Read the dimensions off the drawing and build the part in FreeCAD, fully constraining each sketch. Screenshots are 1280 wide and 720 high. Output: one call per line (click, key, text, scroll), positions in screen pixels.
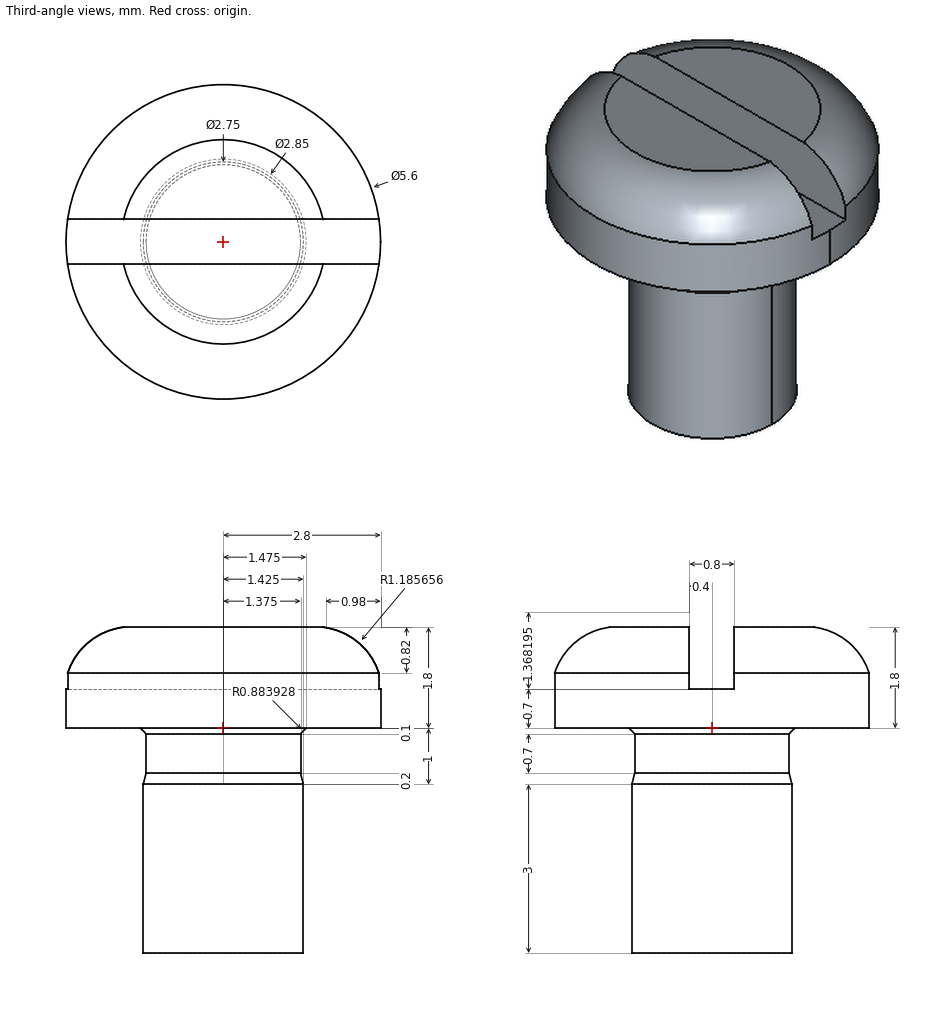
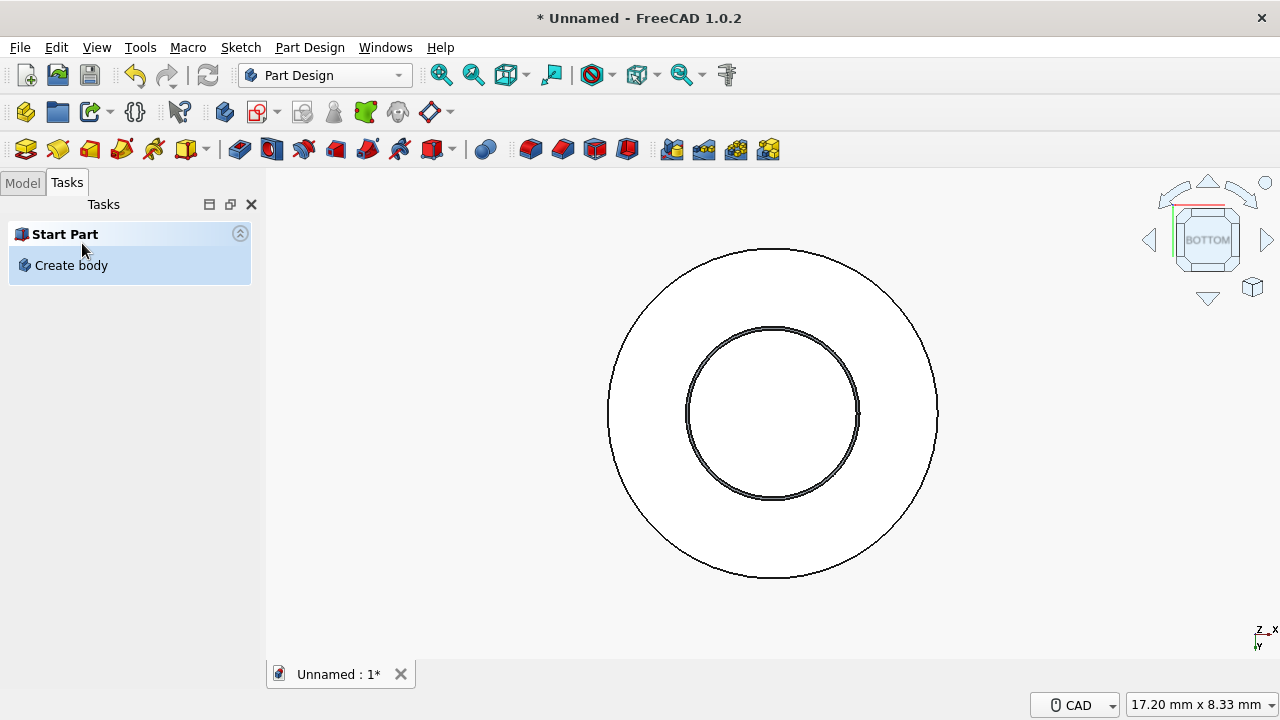
click(773, 412)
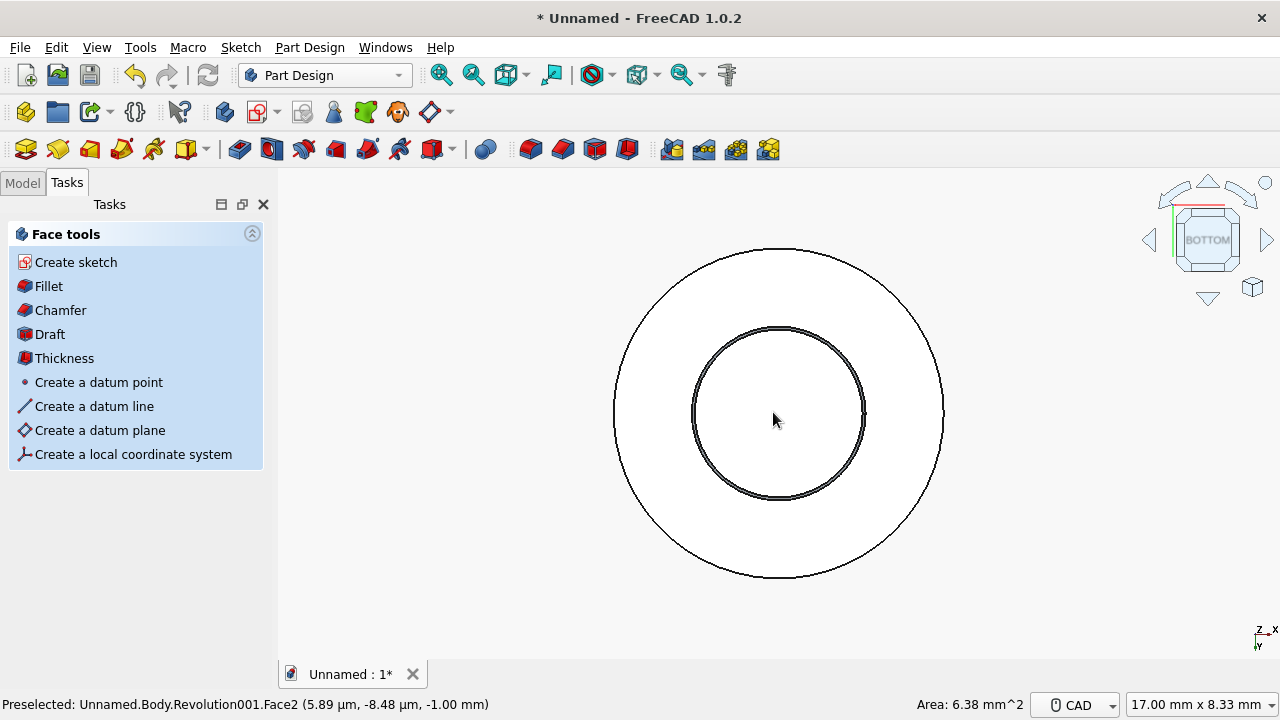
click(258, 112)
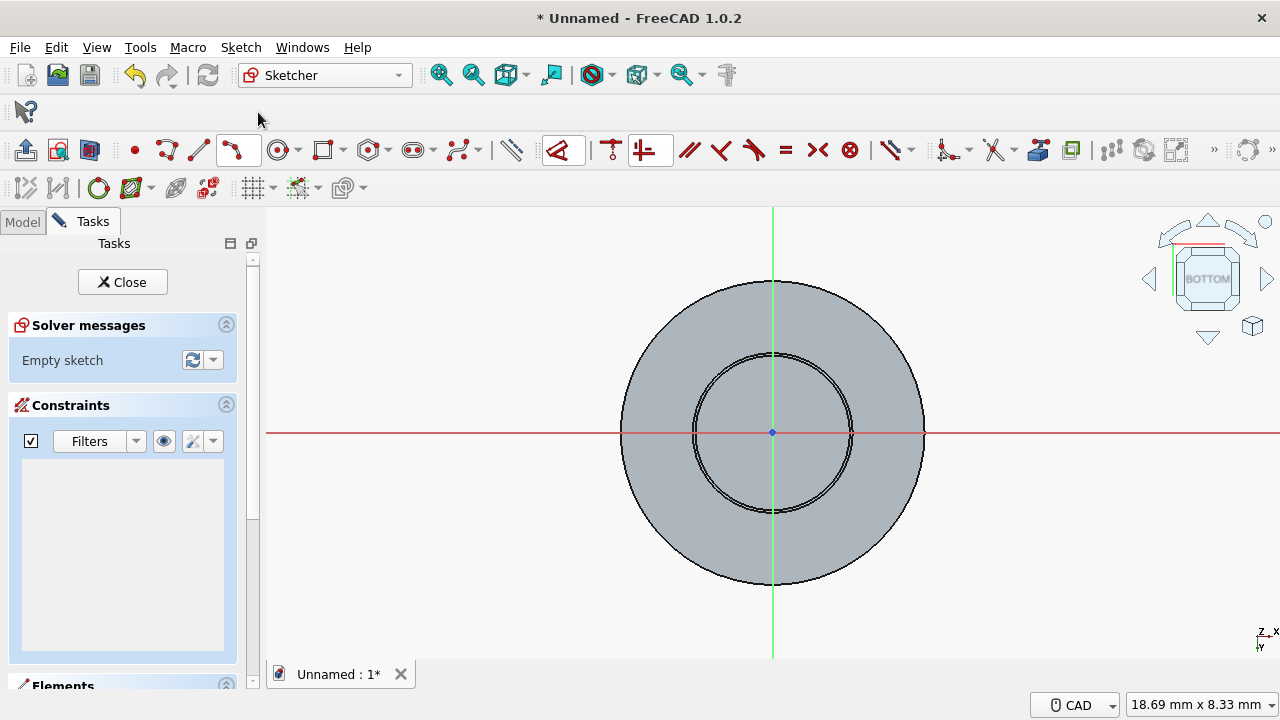
scroll(856, 433, up, 3)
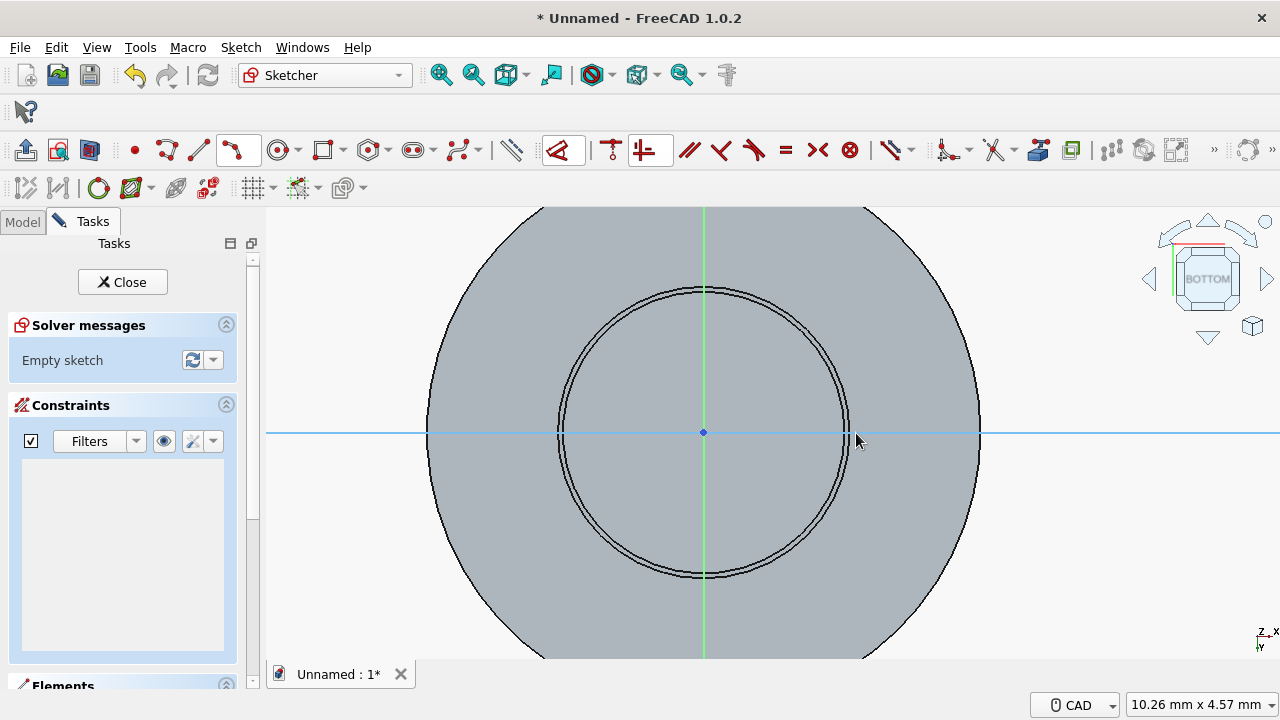
click(278, 150)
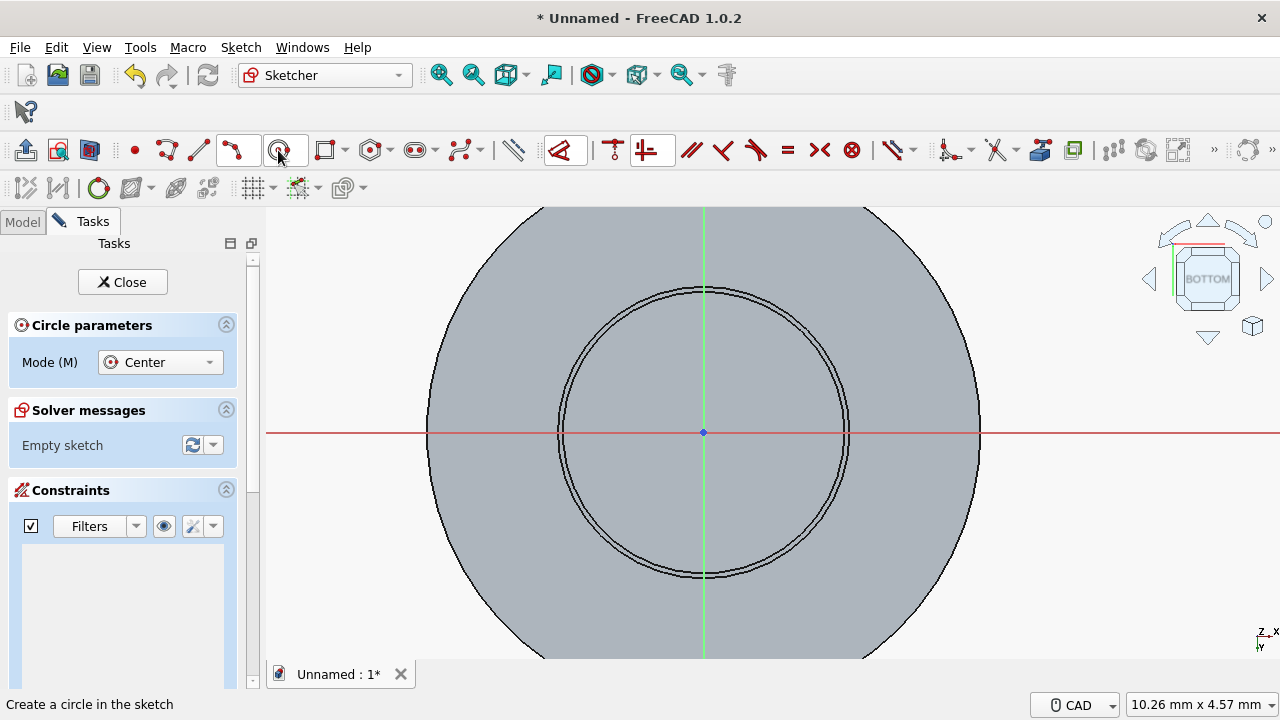
click(704, 433)
click(803, 333)
key(Escape)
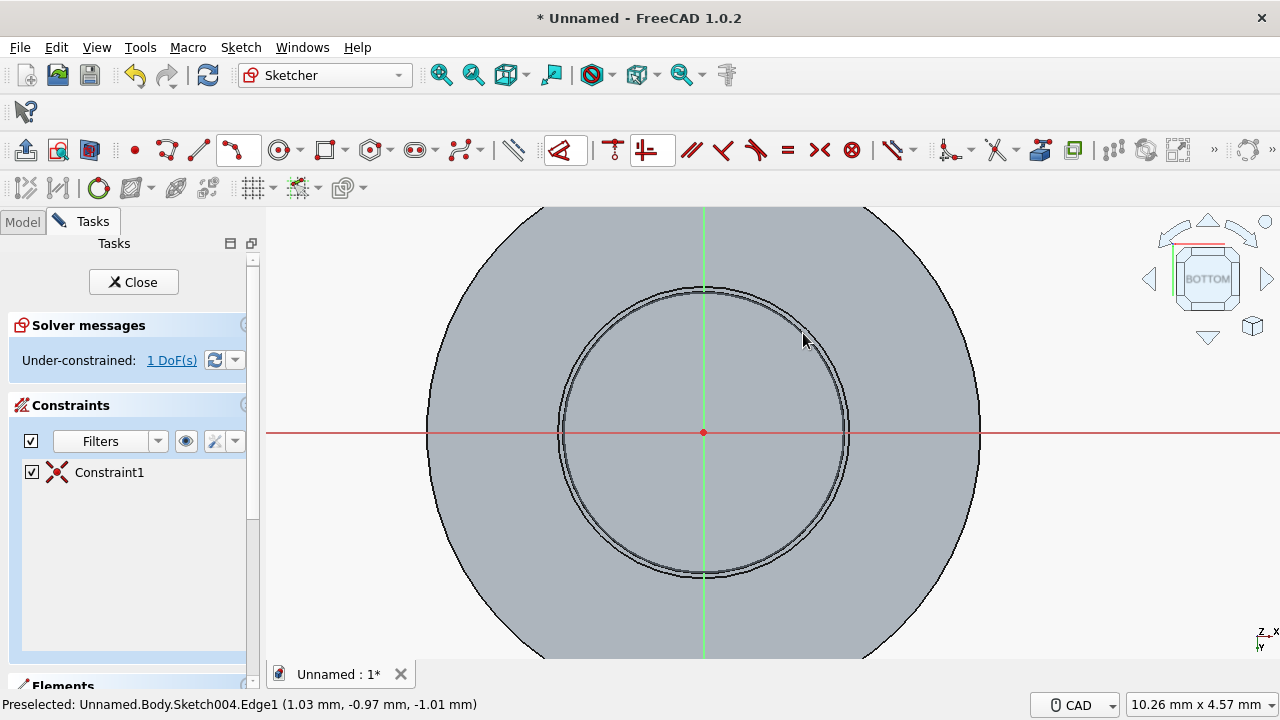
click(802, 333)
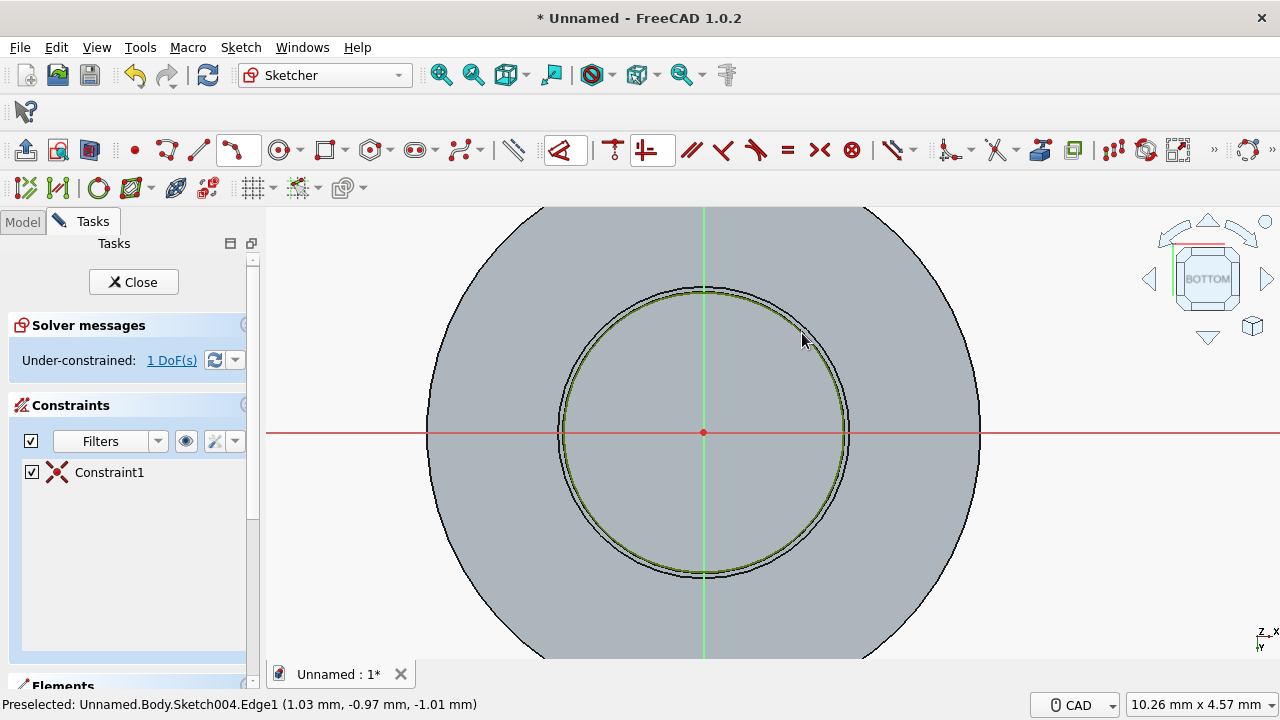
key(k)
key(o)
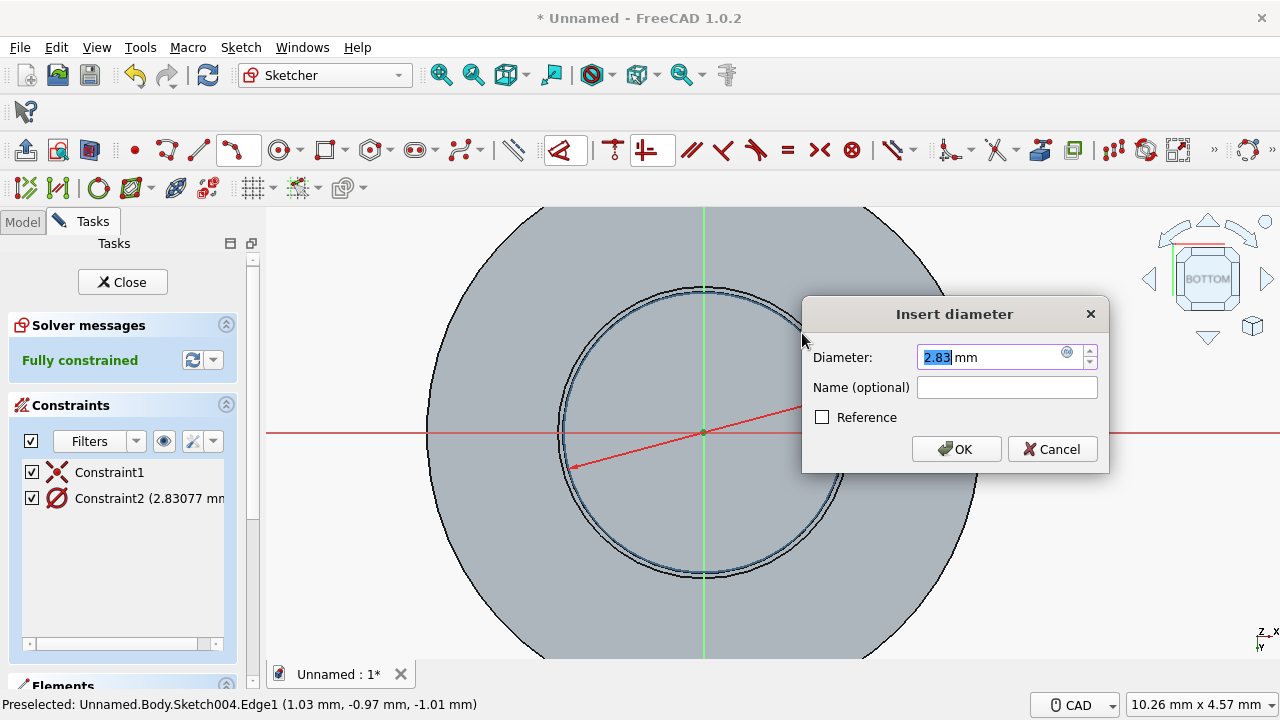
text(2.85)
key(Return)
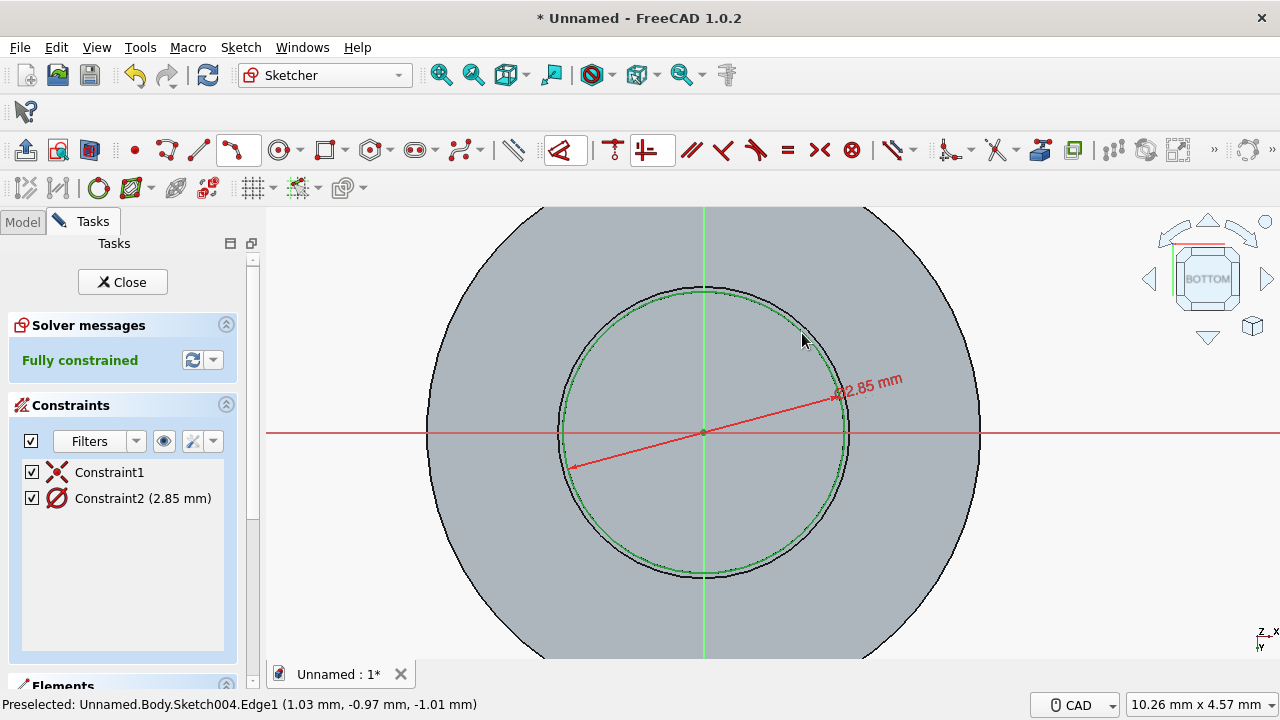
click(123, 282)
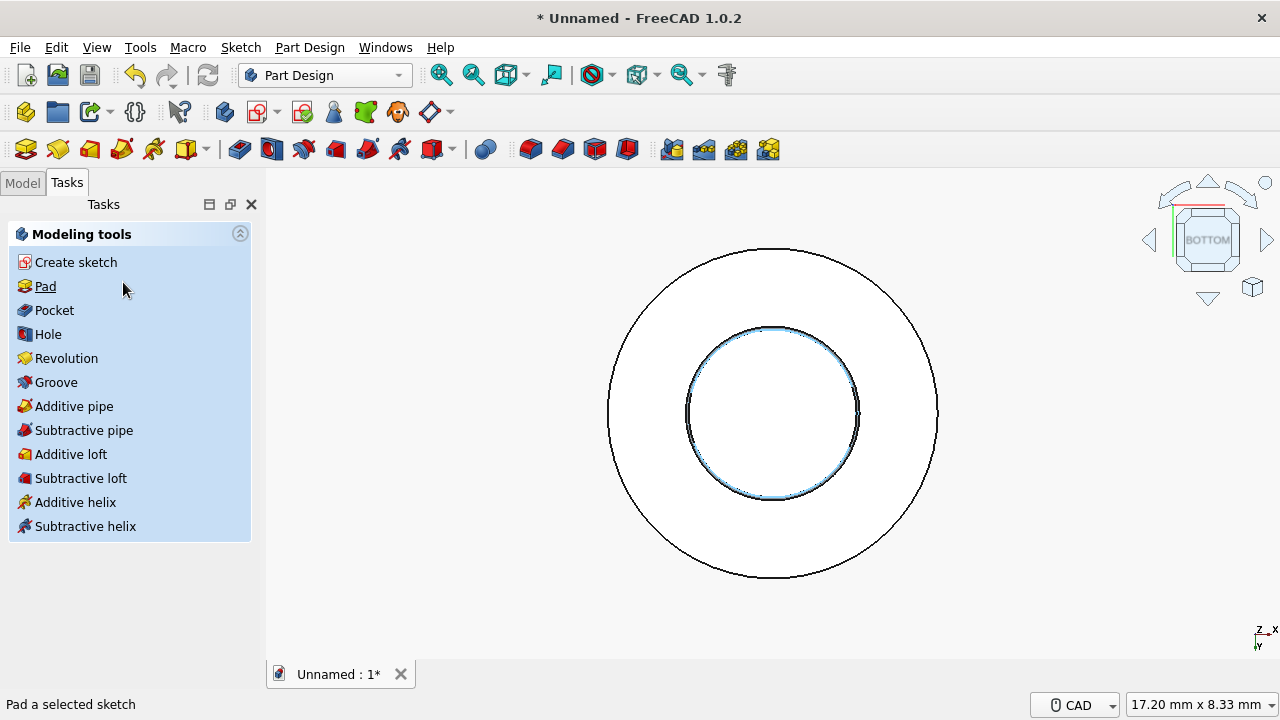
click(26, 150)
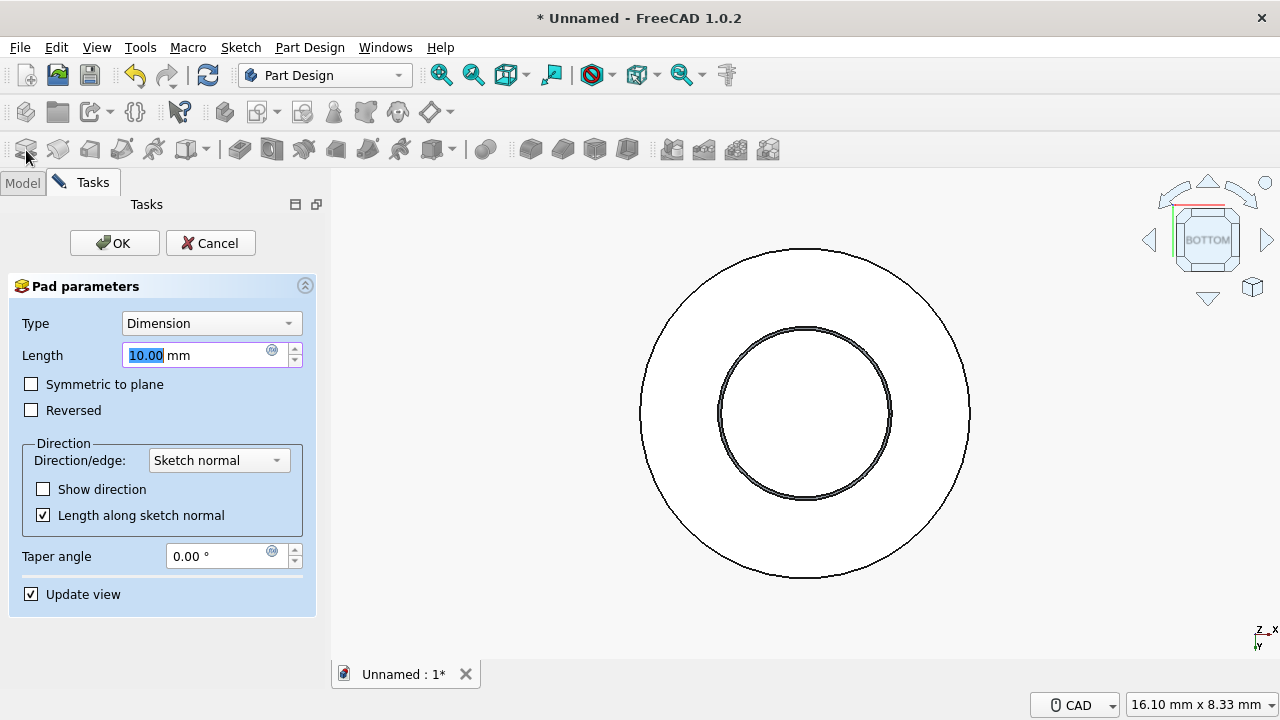
text(3)
key(Tab)